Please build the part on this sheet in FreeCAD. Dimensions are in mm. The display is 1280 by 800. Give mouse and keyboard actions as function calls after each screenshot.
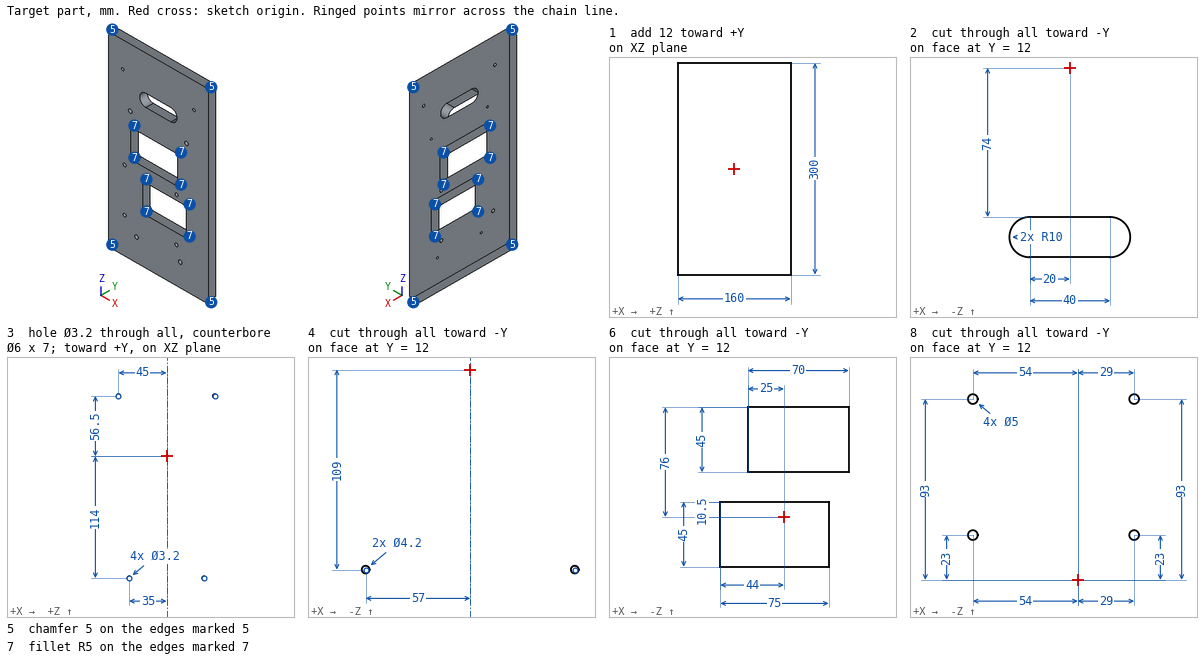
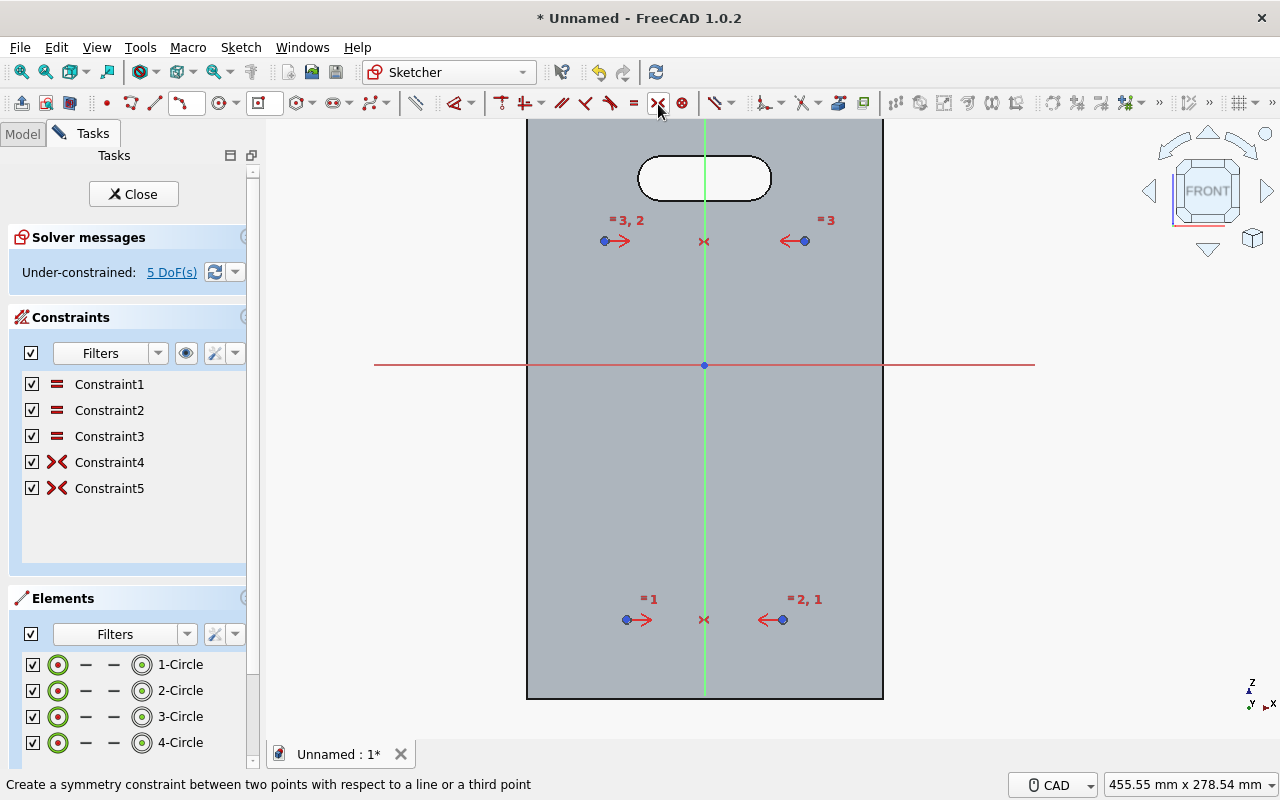
click(454, 104)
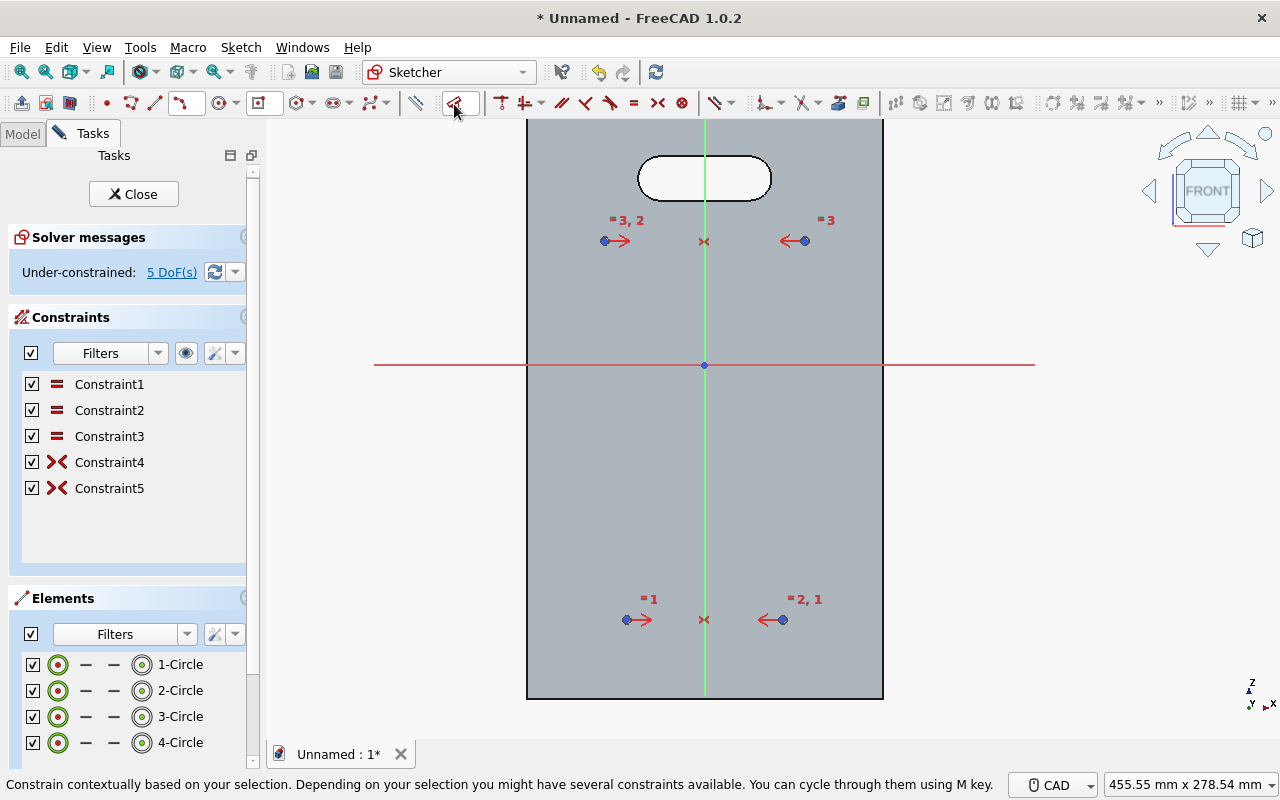
scroll(627, 616, up, 9)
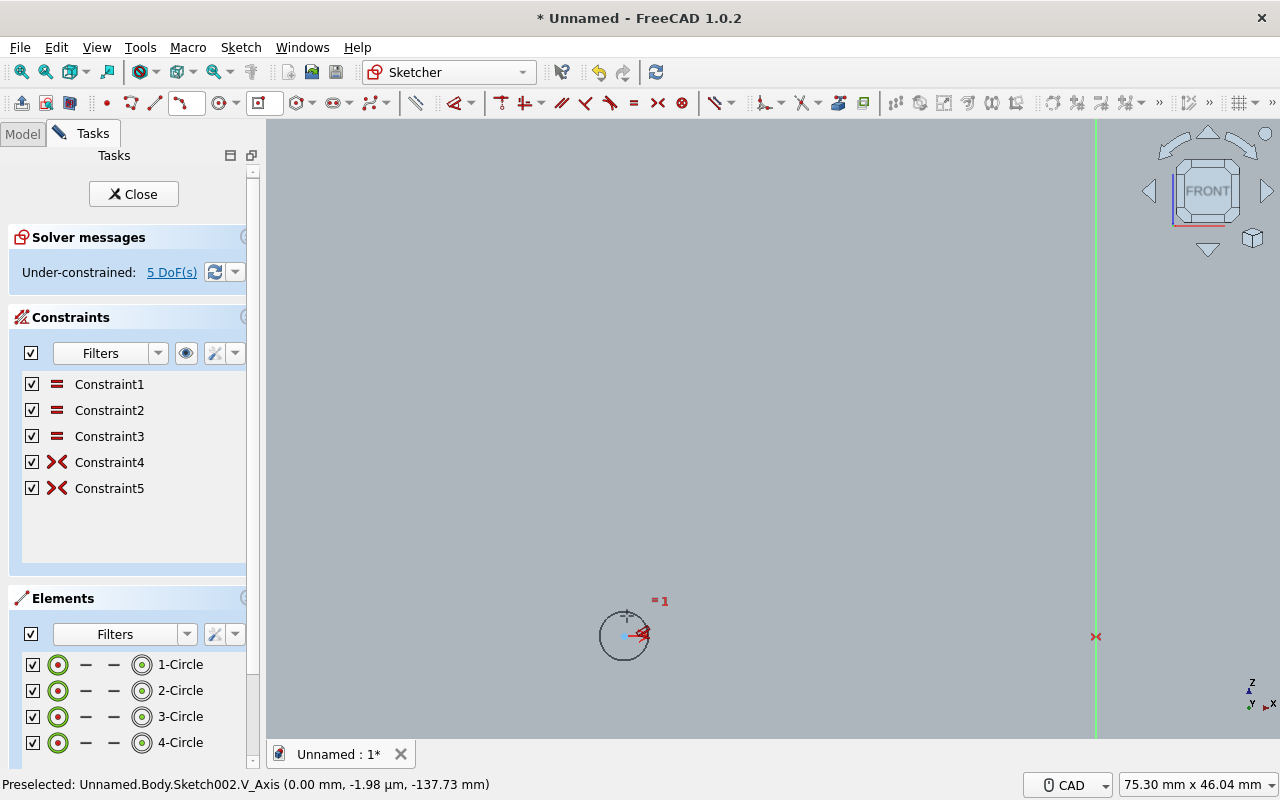
click(625, 612)
click(626, 580)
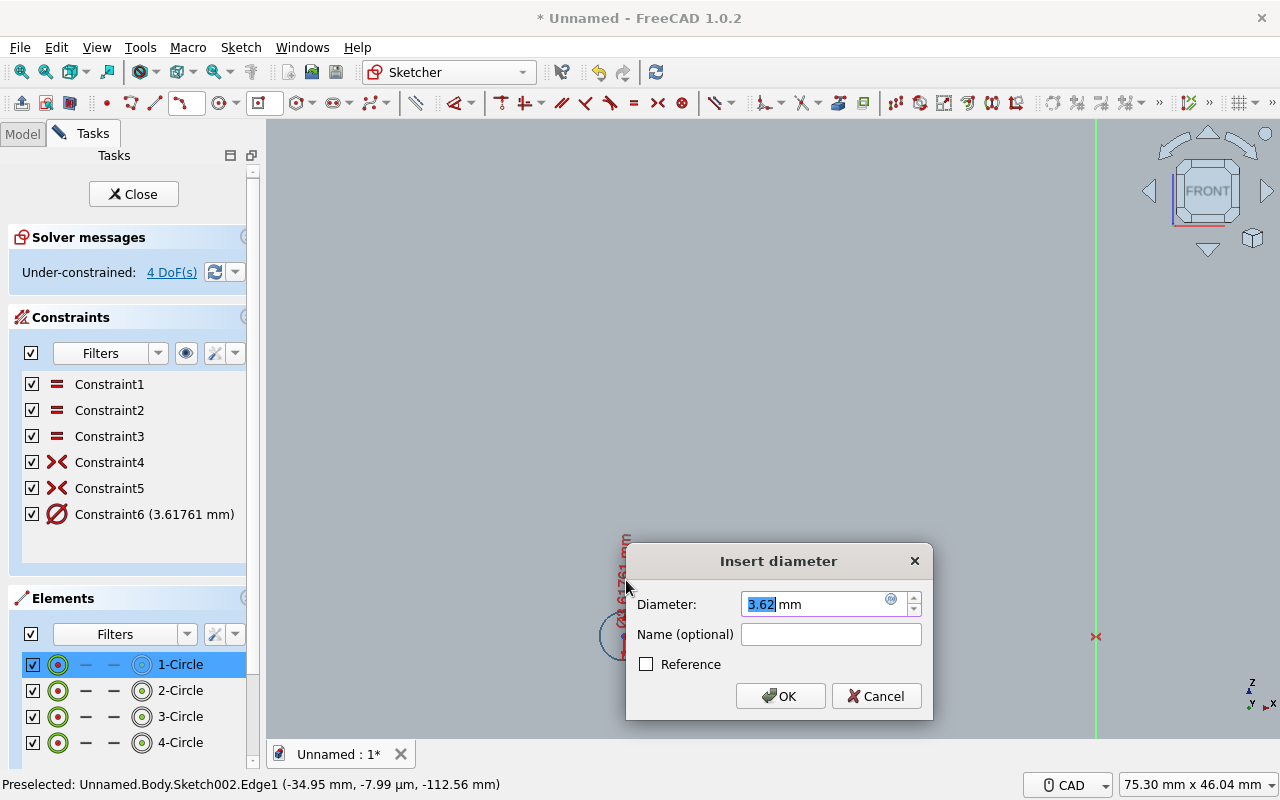
text(3.2)
key(Return)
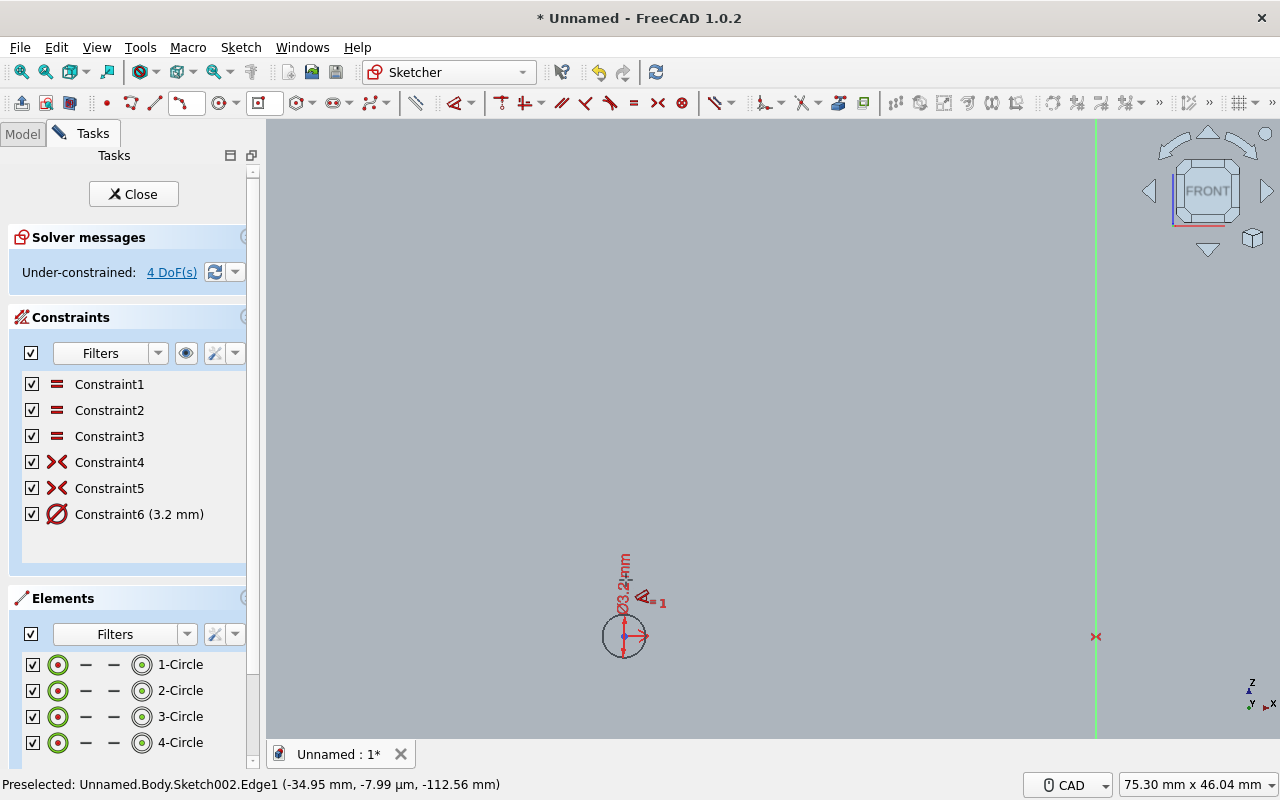
scroll(627, 616, down, 9)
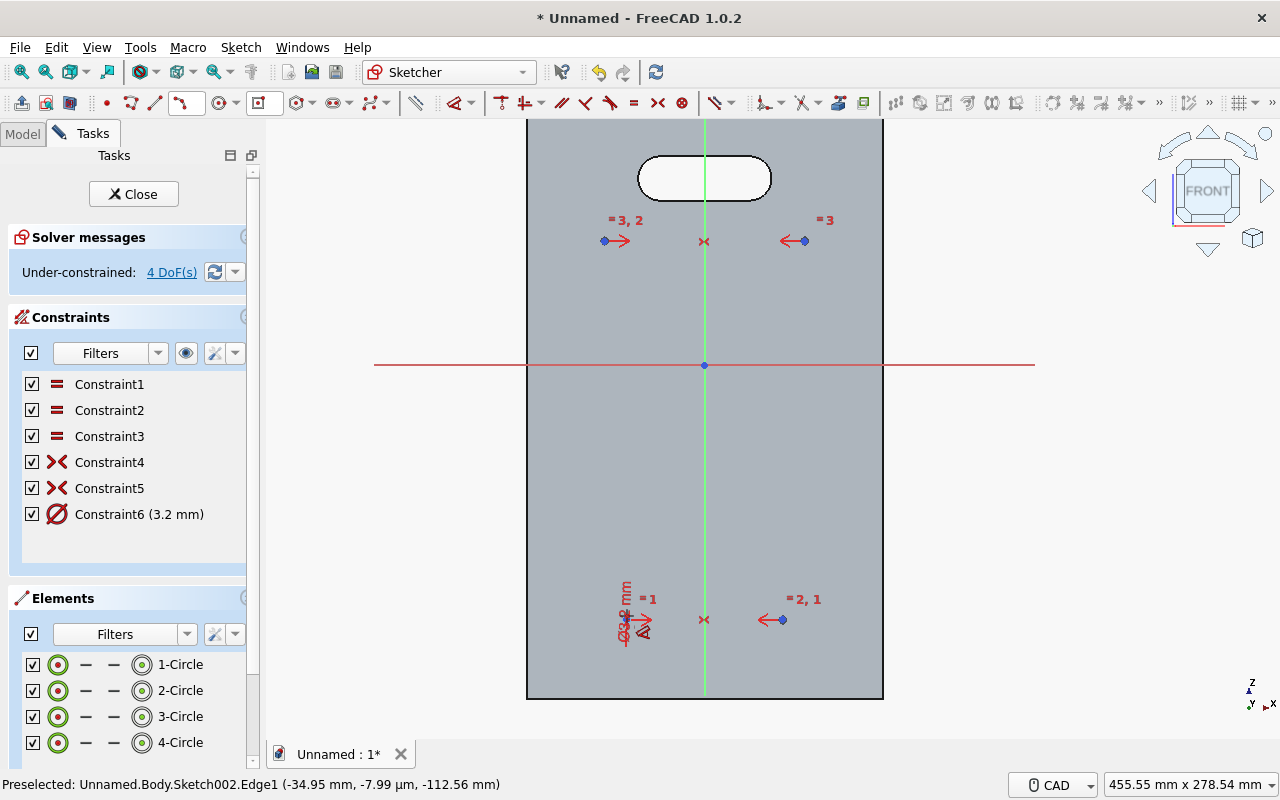
click(627, 620)
click(666, 654)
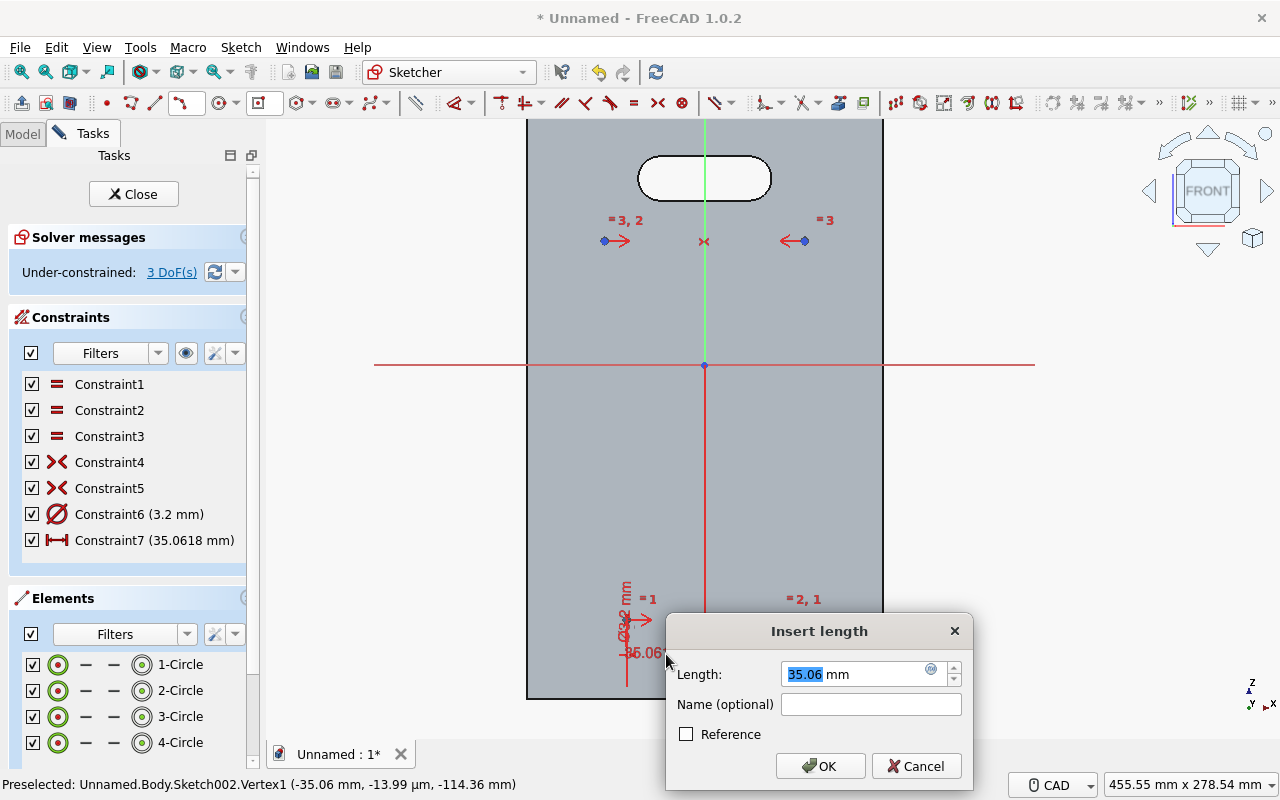
text(35)
key(Return)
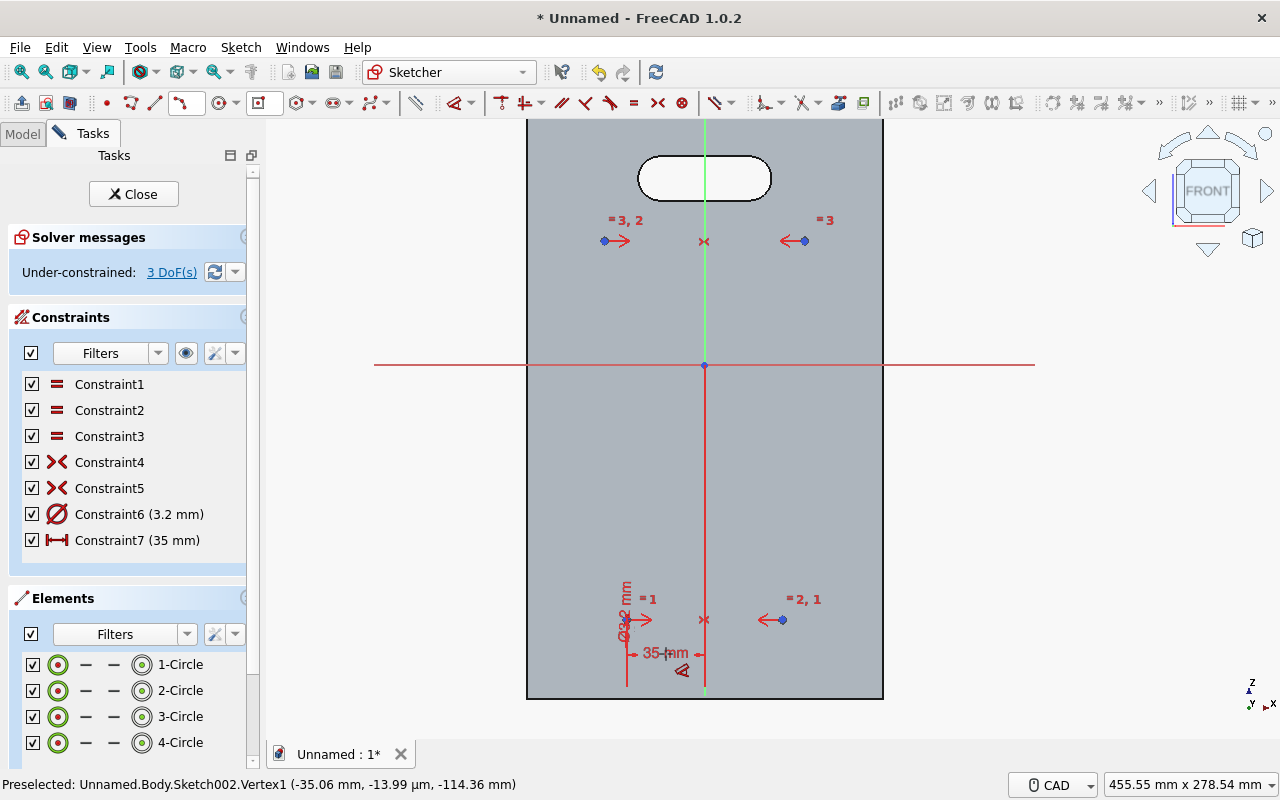
click(605, 241)
click(655, 207)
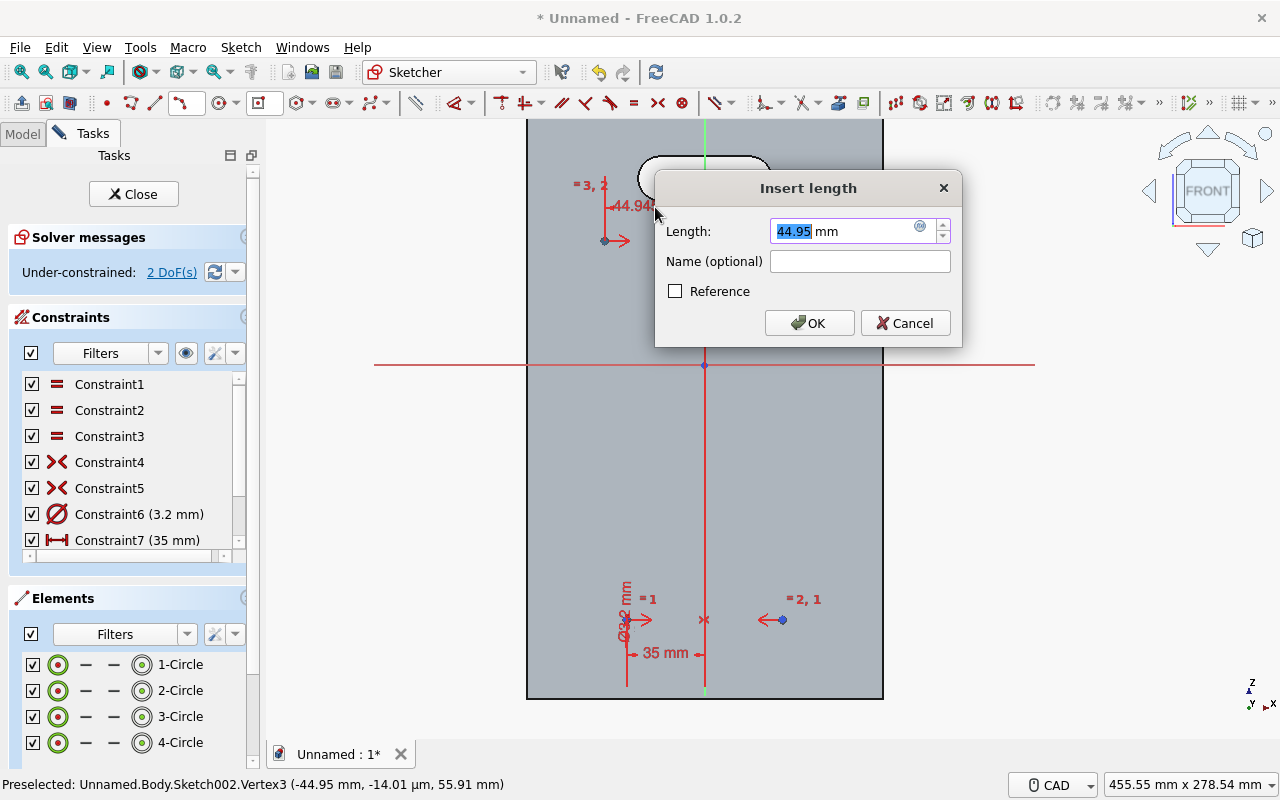
text(45)
key(Return)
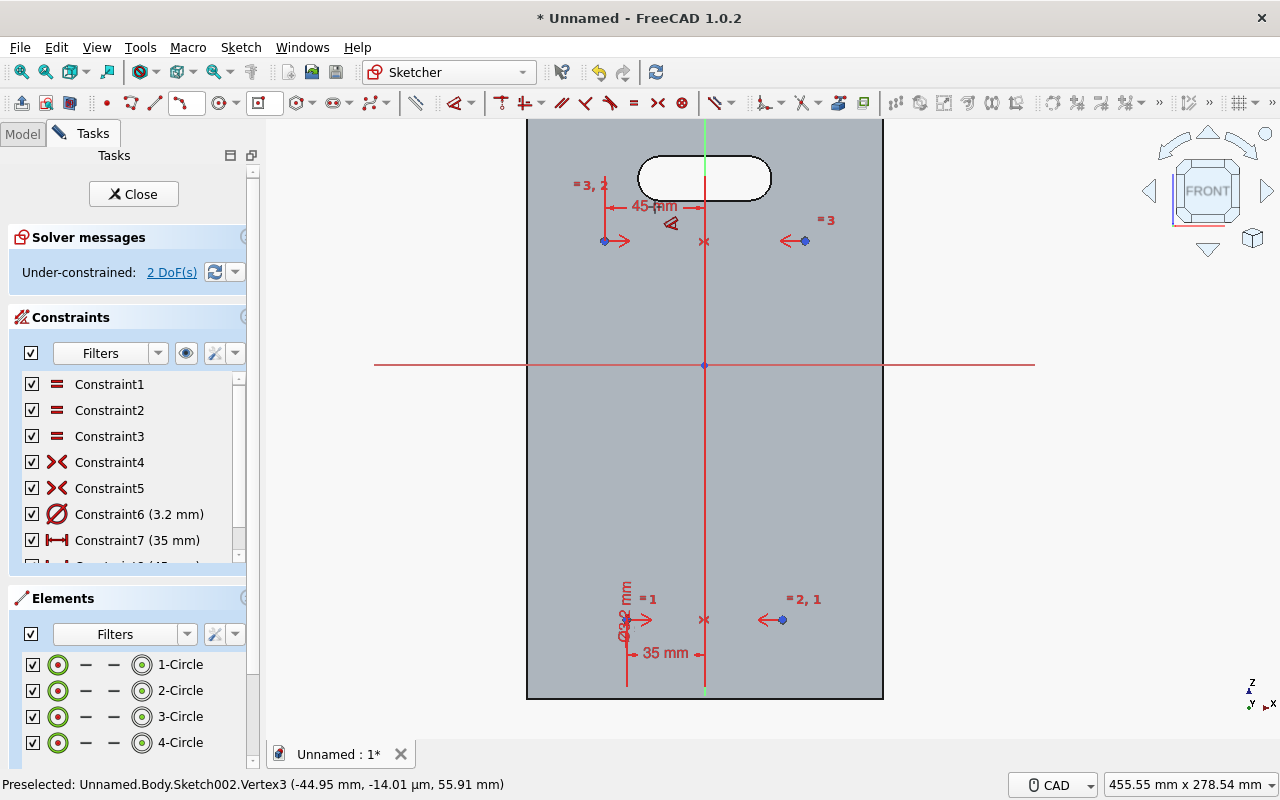
click(627, 620)
click(593, 493)